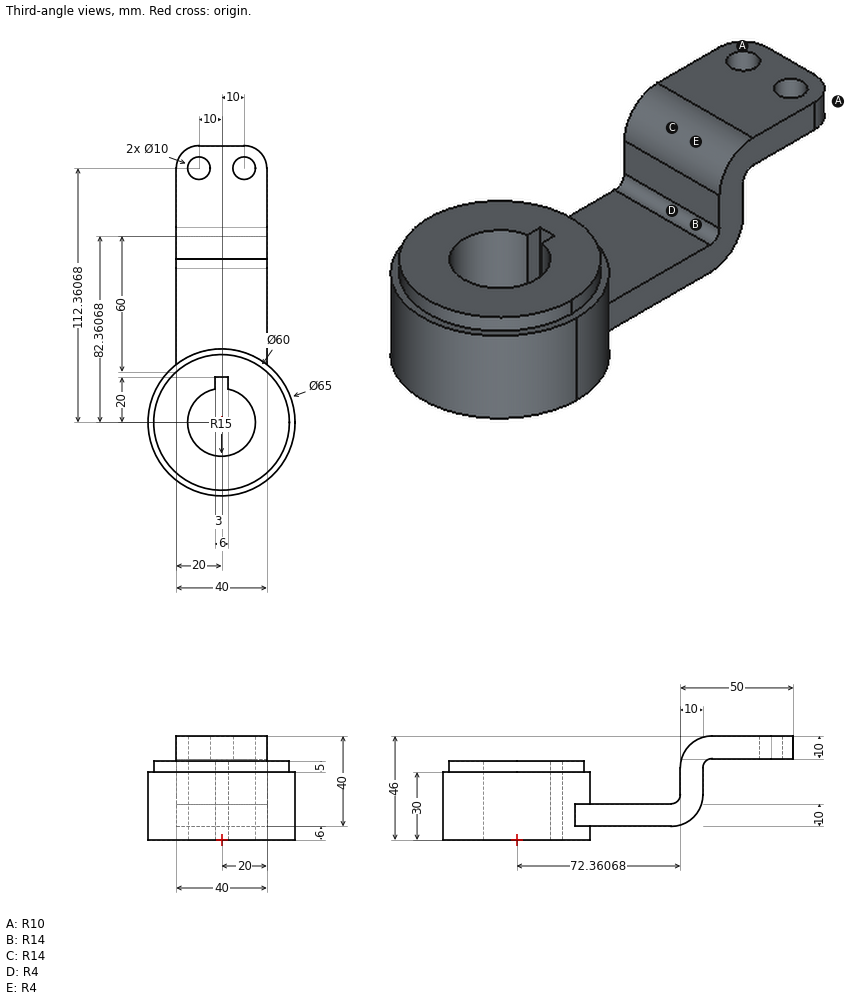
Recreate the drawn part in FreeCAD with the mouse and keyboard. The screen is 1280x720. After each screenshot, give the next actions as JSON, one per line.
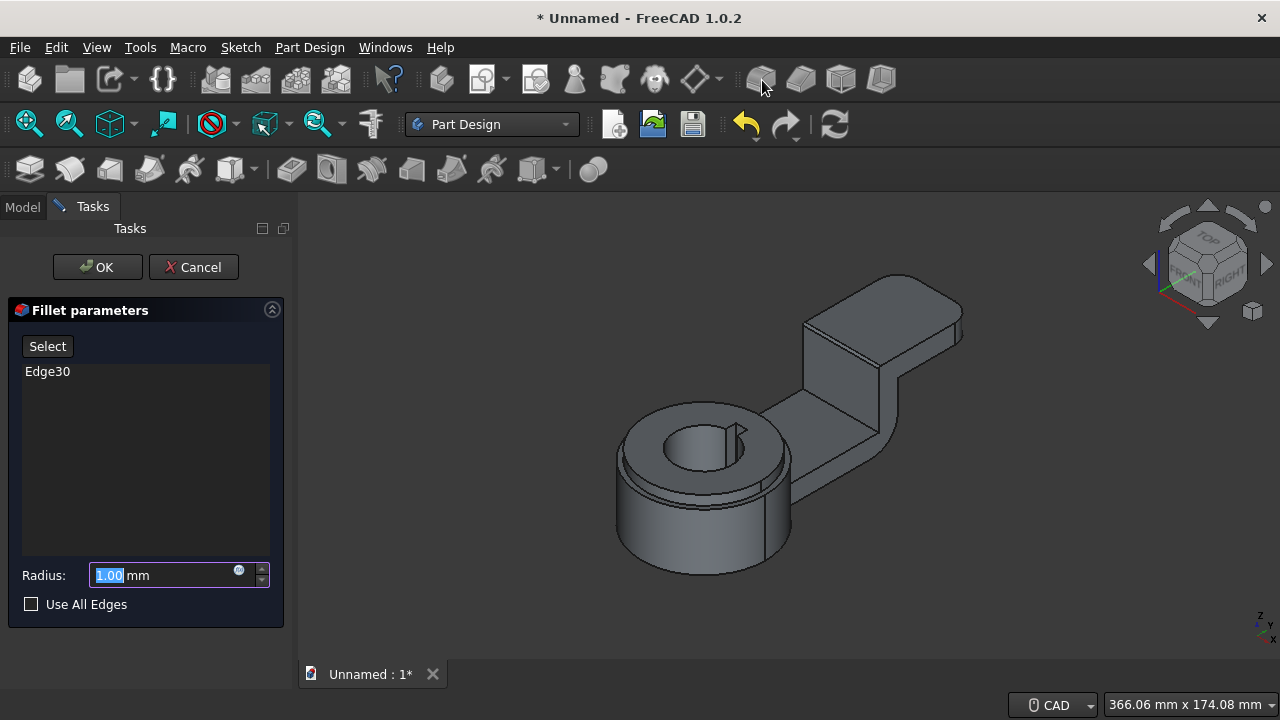
{"action": "type", "text": "14"}
{"action": "key", "text": "Tab"}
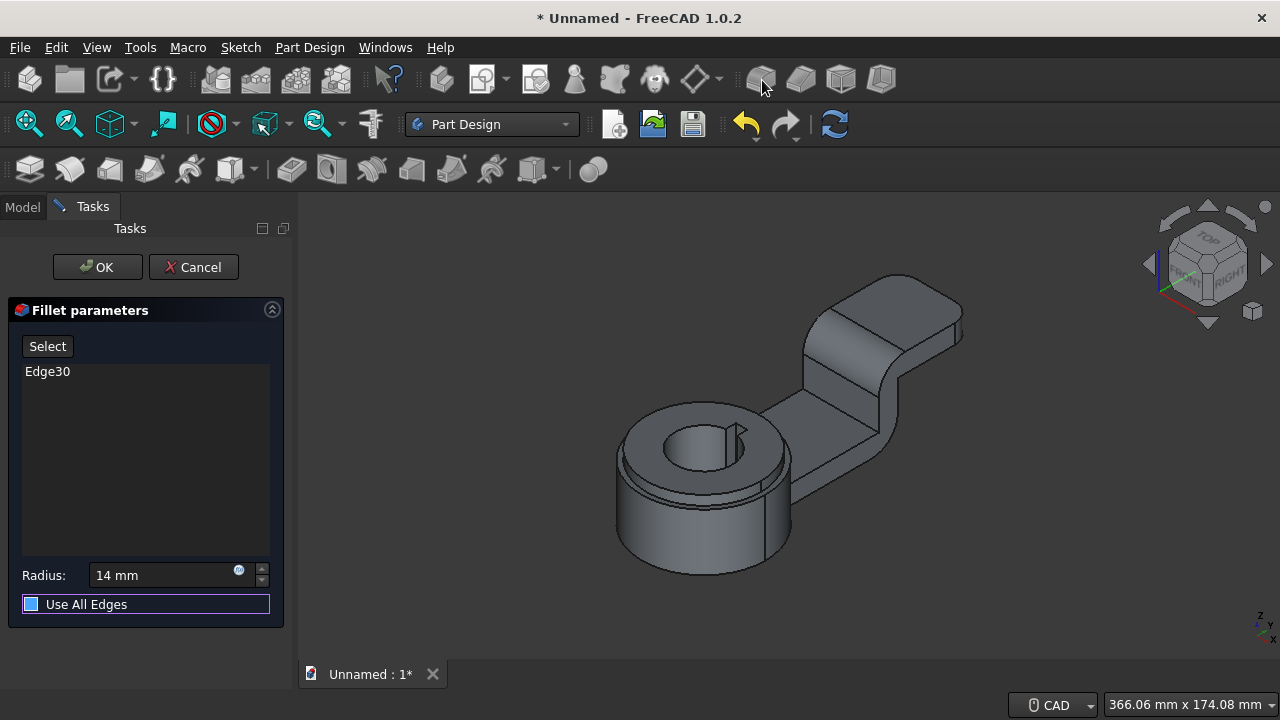
{"action": "left_click", "coordinate": [98, 267]}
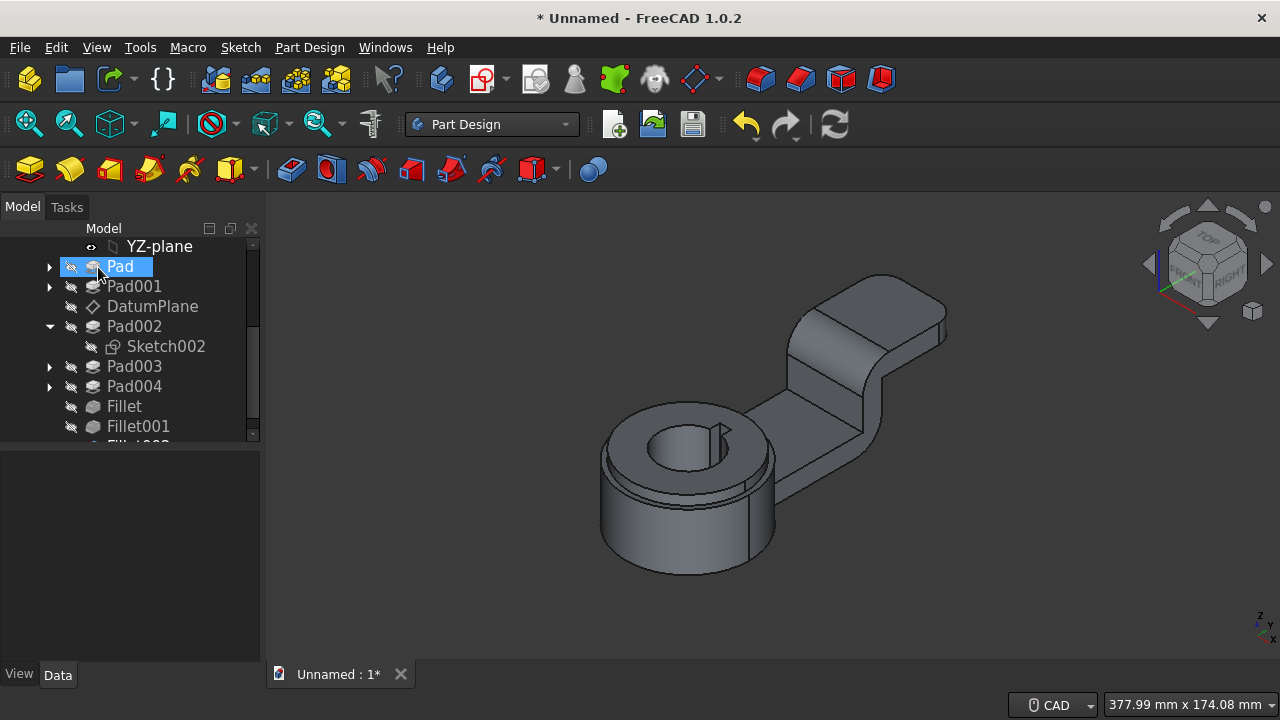
{"action": "key", "text": "2"}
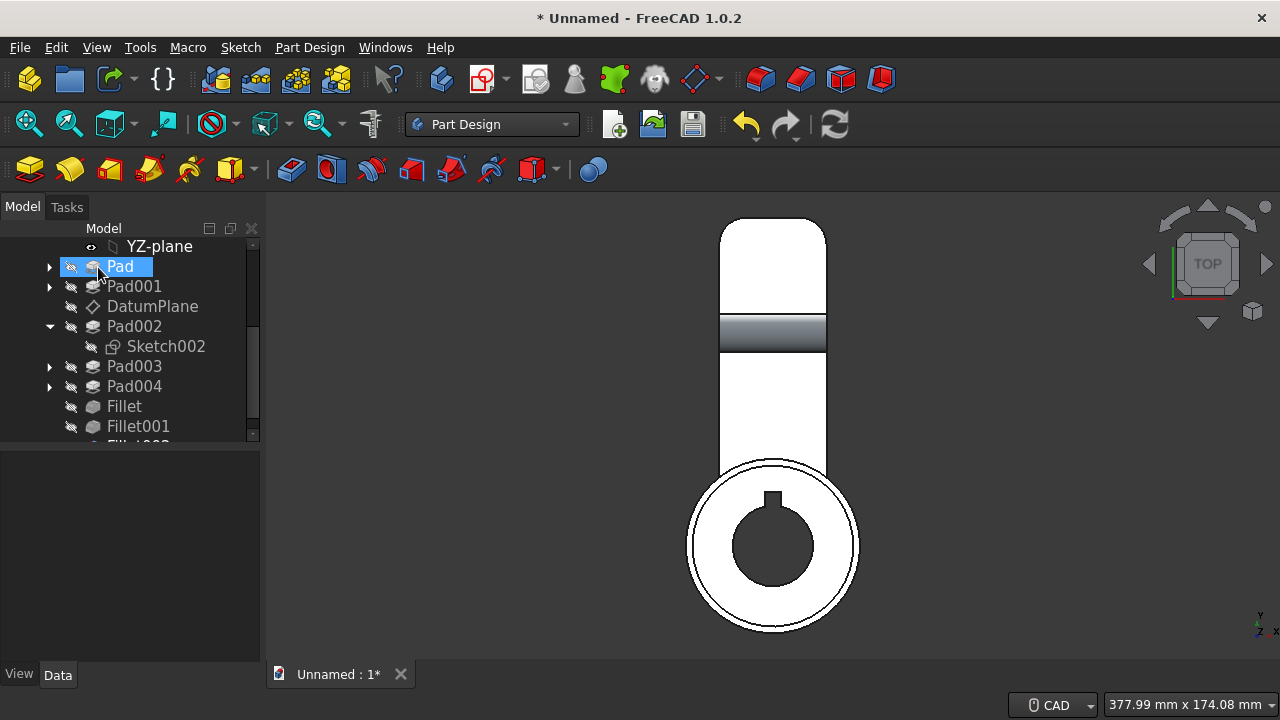
{"action": "key", "text": "0"}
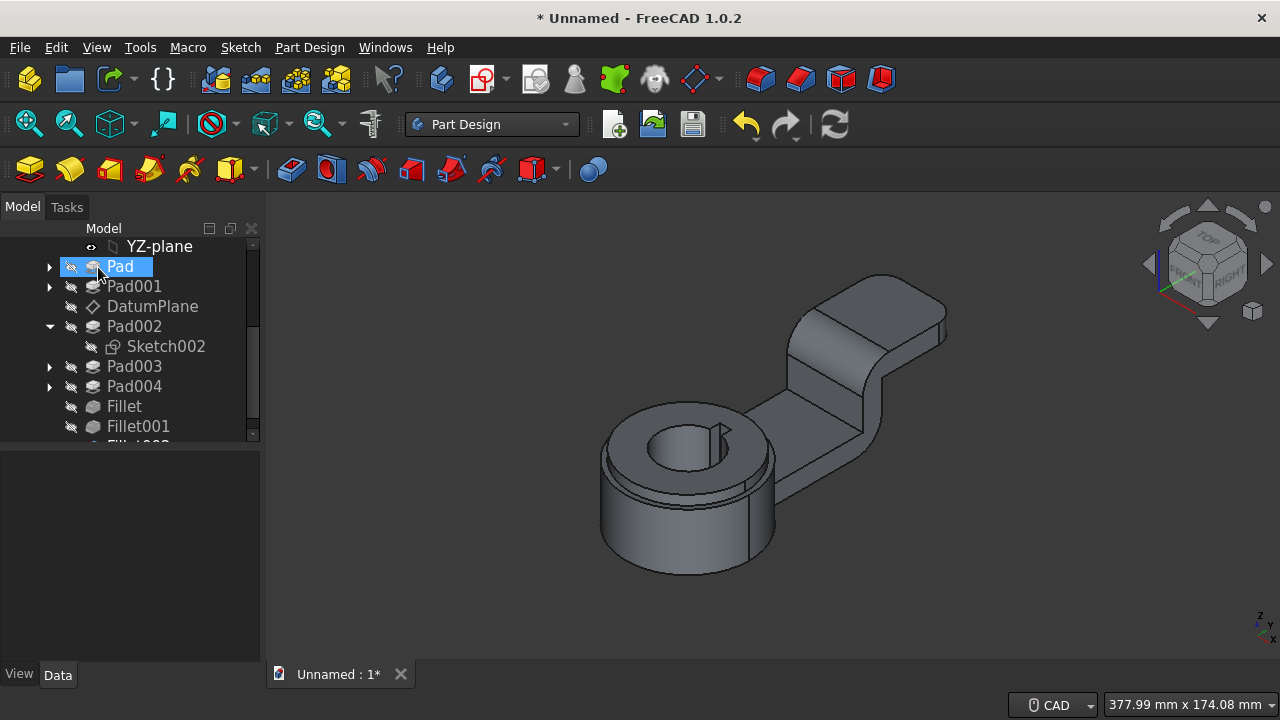
{"action": "key", "text": "1"}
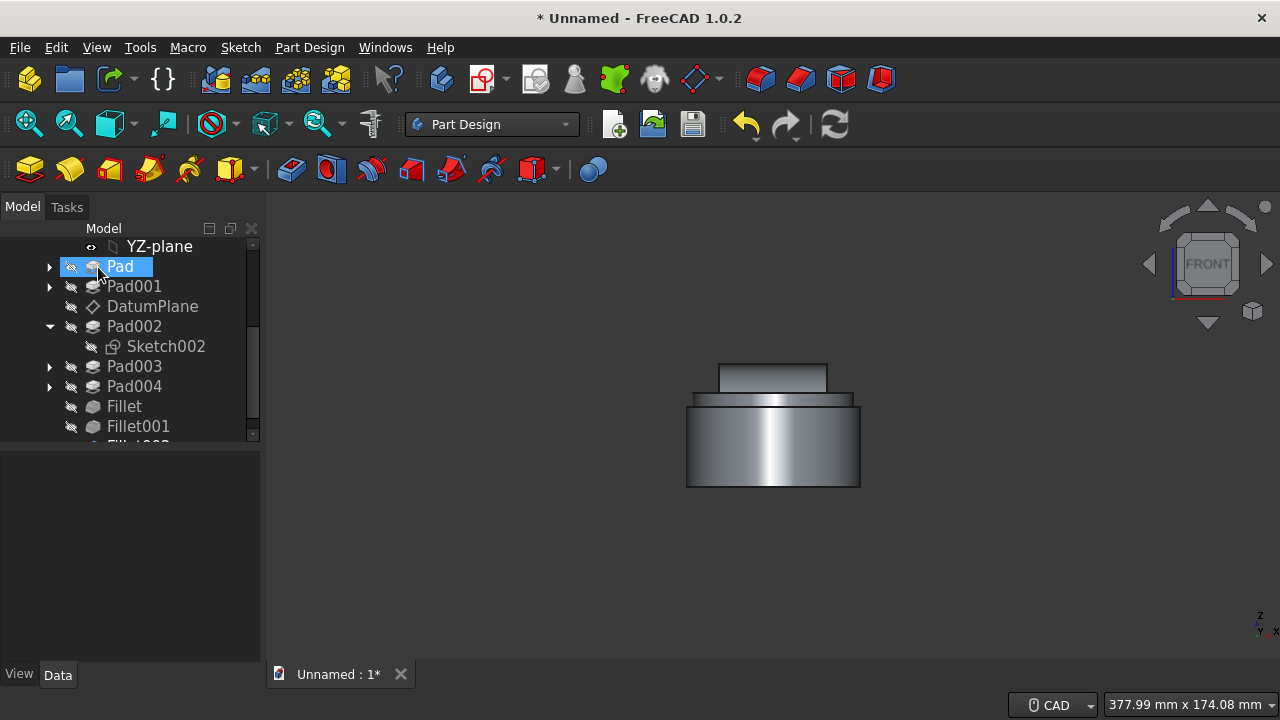
{"action": "key", "text": "v f"}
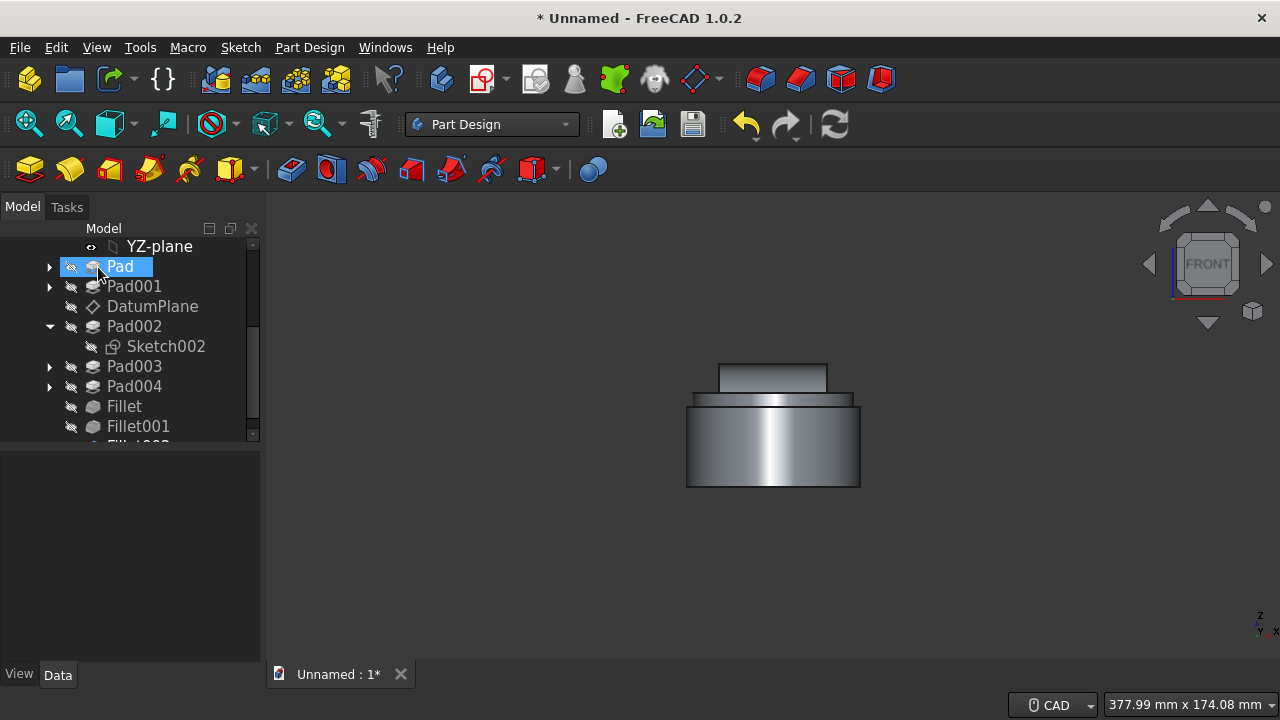
{"action": "key", "text": "3"}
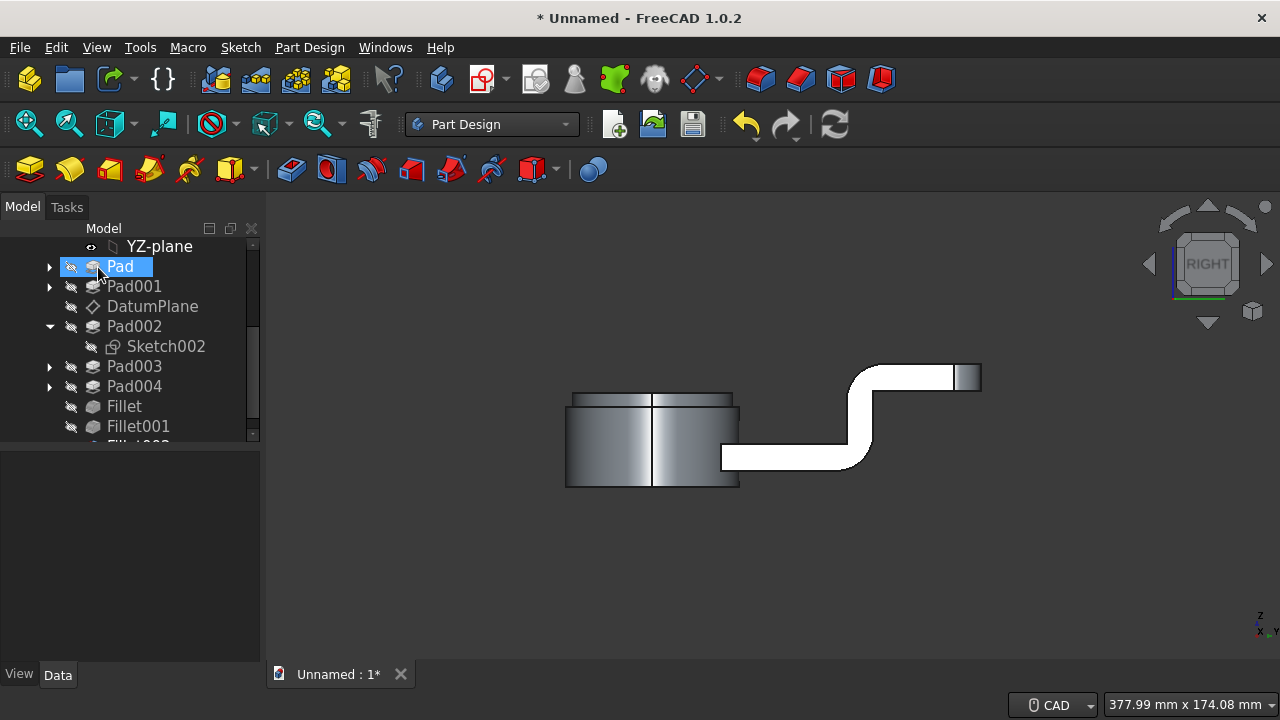
{"action": "left_click", "coordinate": [30, 124]}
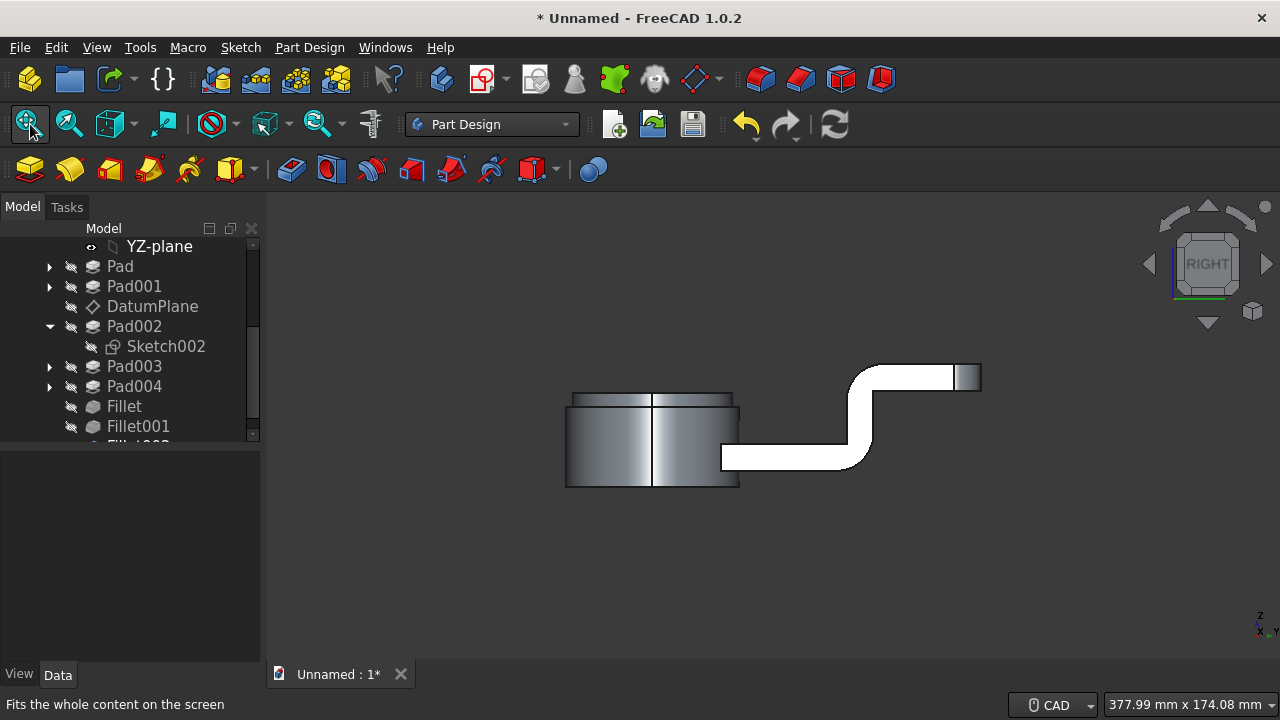
{"action": "key", "text": "5"}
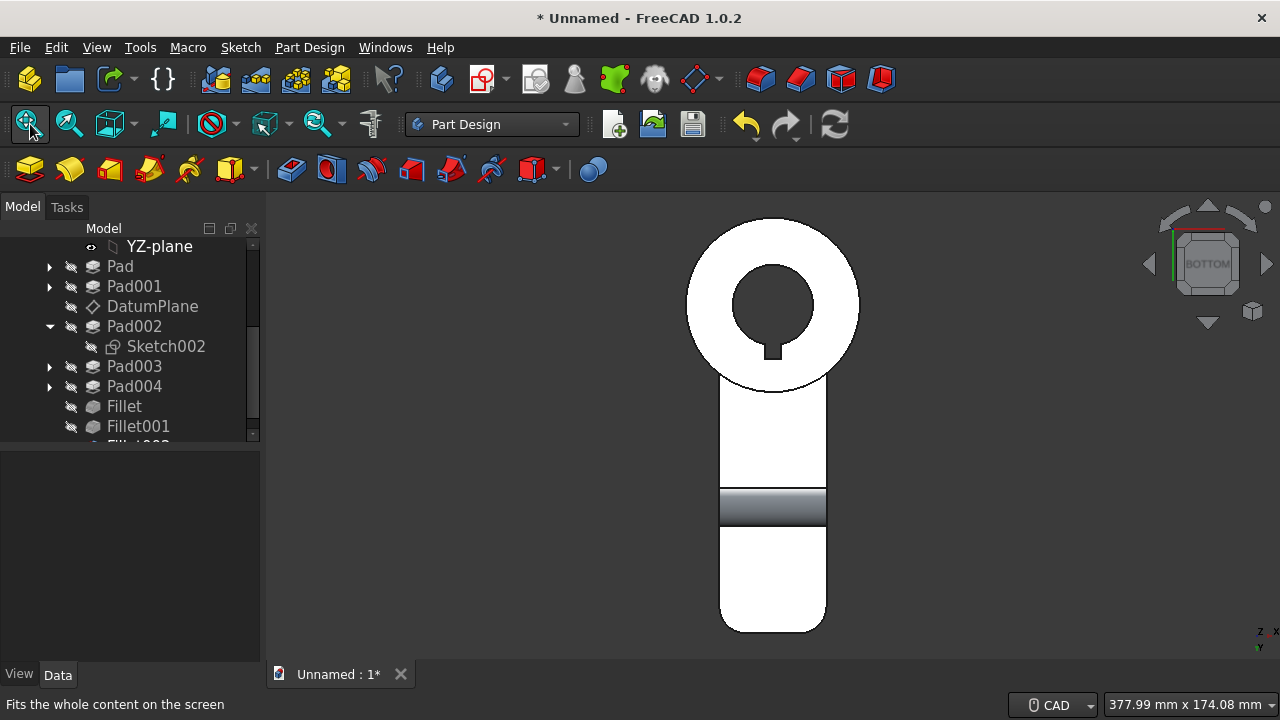
{"action": "key", "text": "4"}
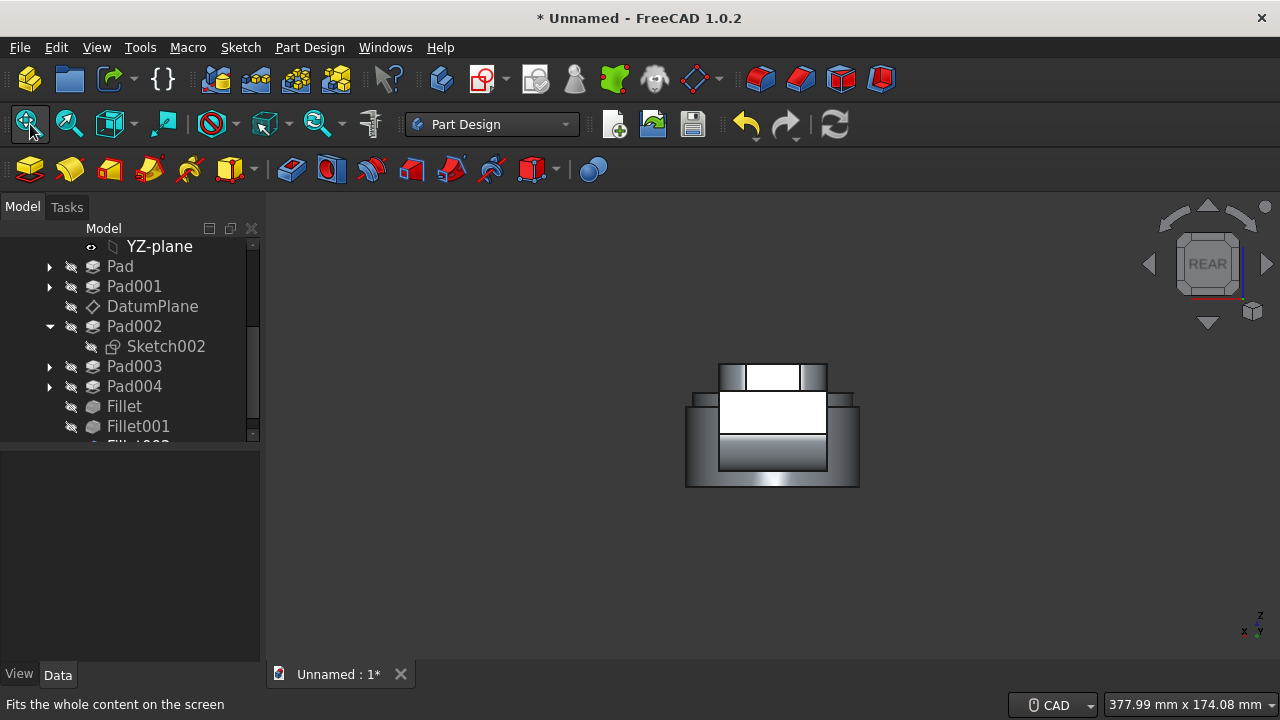
{"action": "left_click", "coordinate": [30, 124]}